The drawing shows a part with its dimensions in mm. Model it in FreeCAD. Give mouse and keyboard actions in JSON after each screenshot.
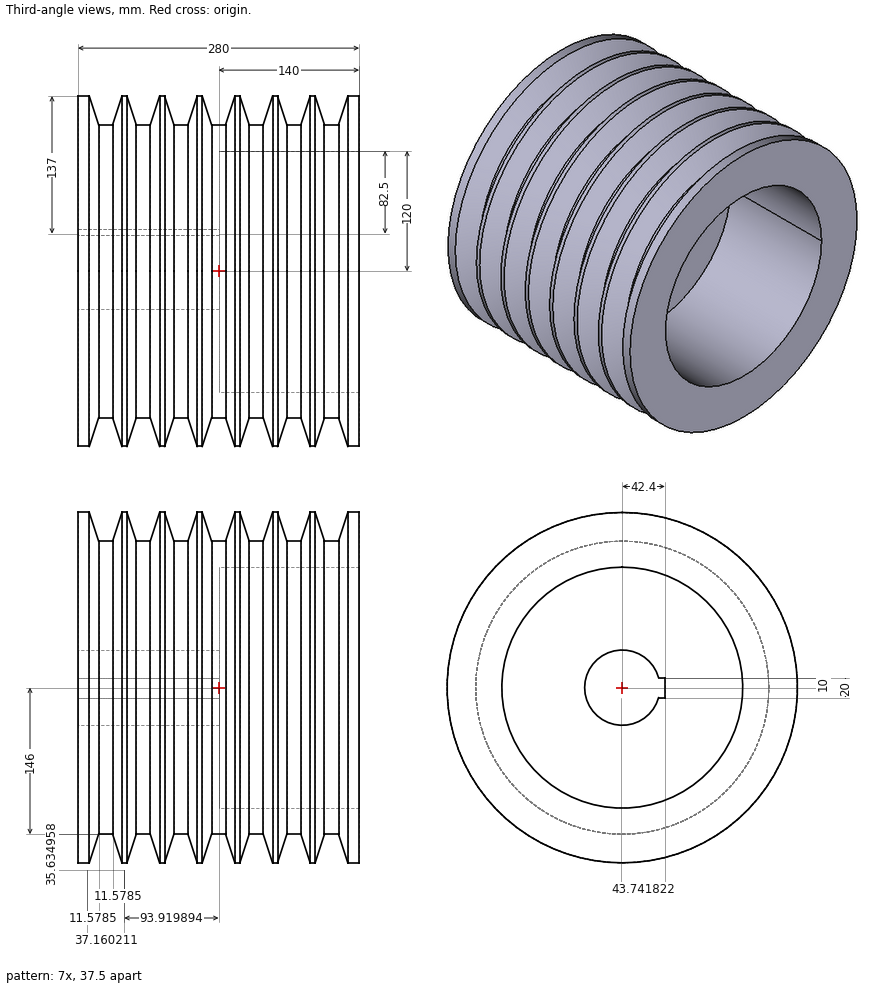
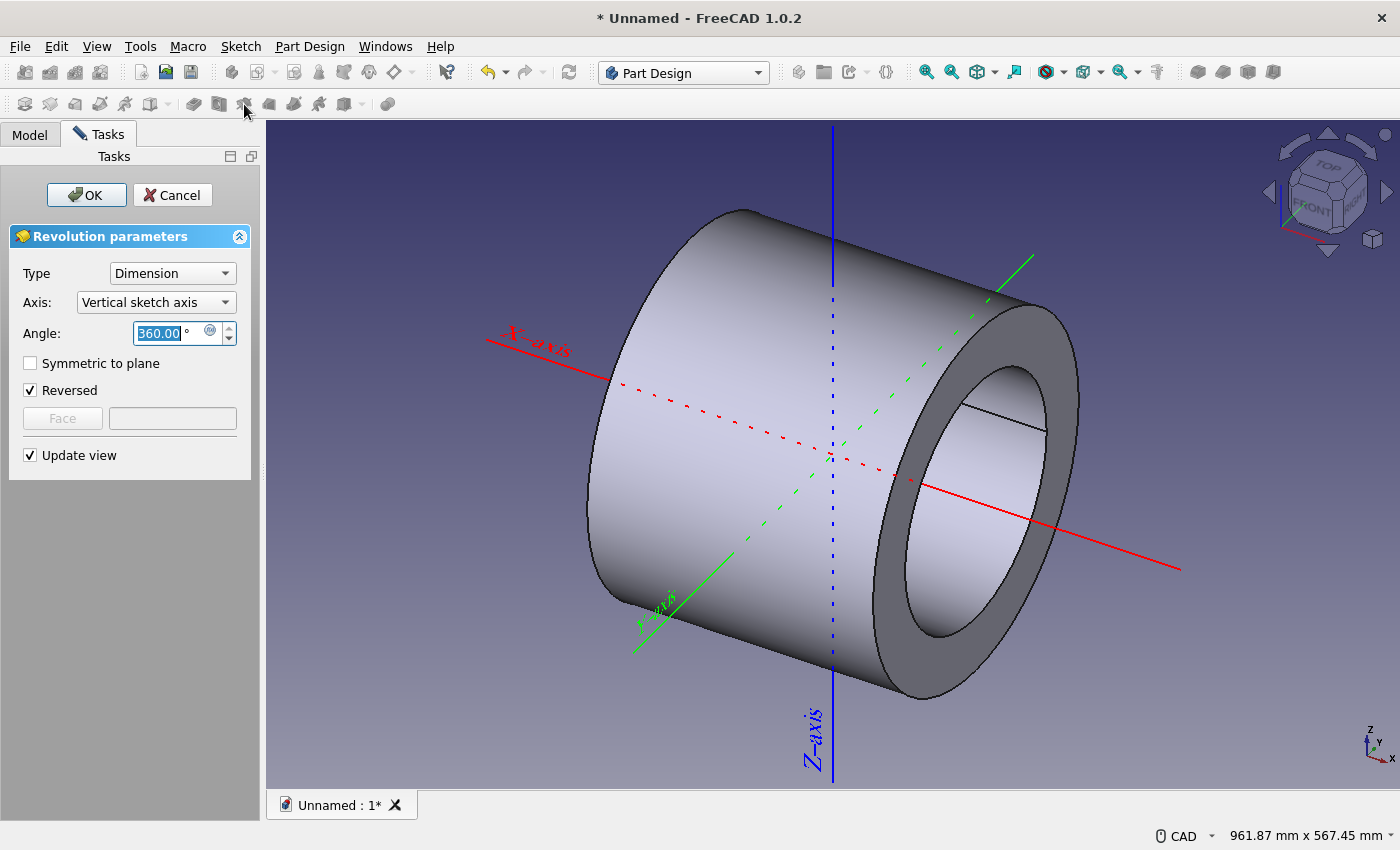
{"action": "left_click", "coordinate": [157, 302]}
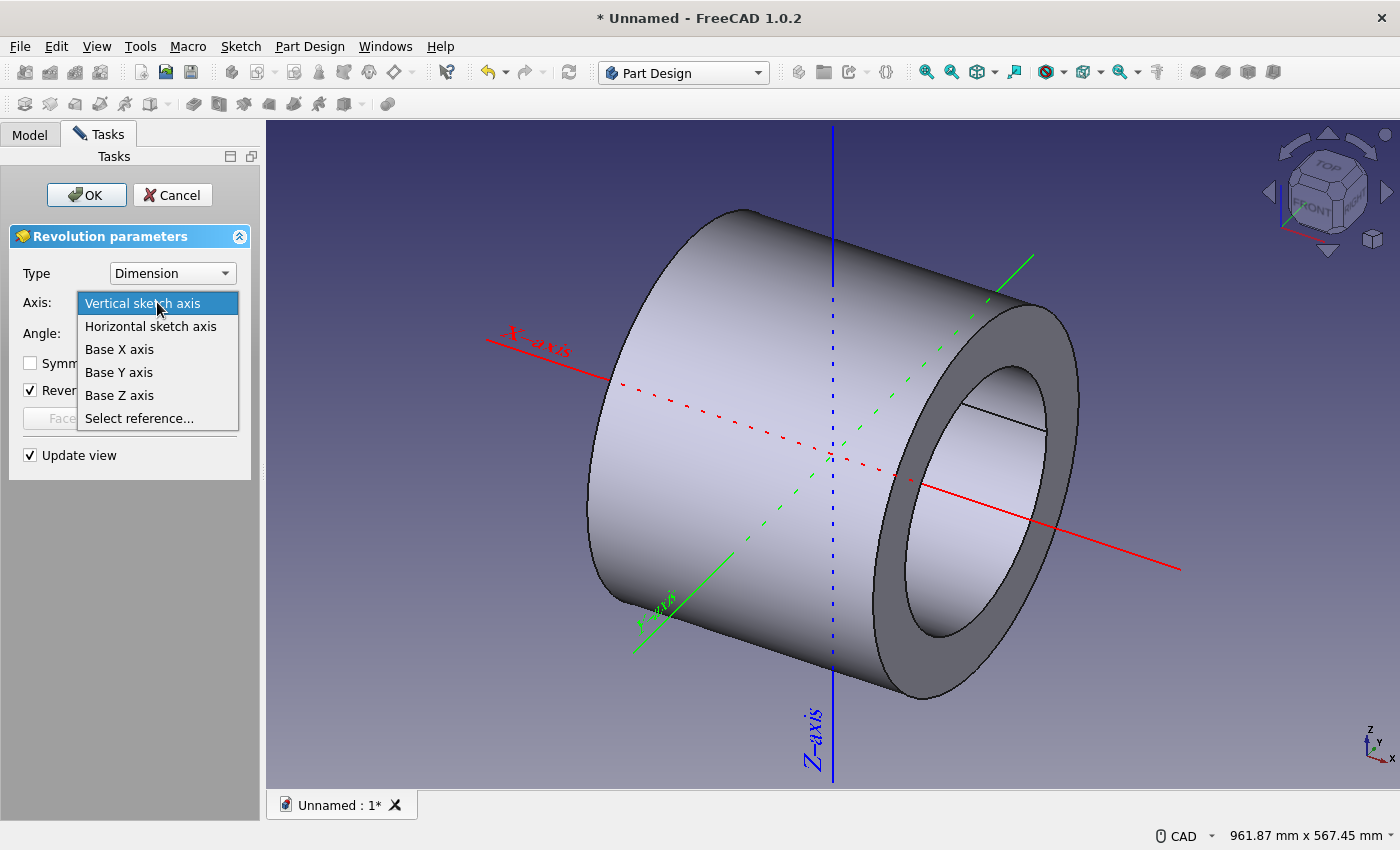
{"action": "left_click", "coordinate": [156, 326]}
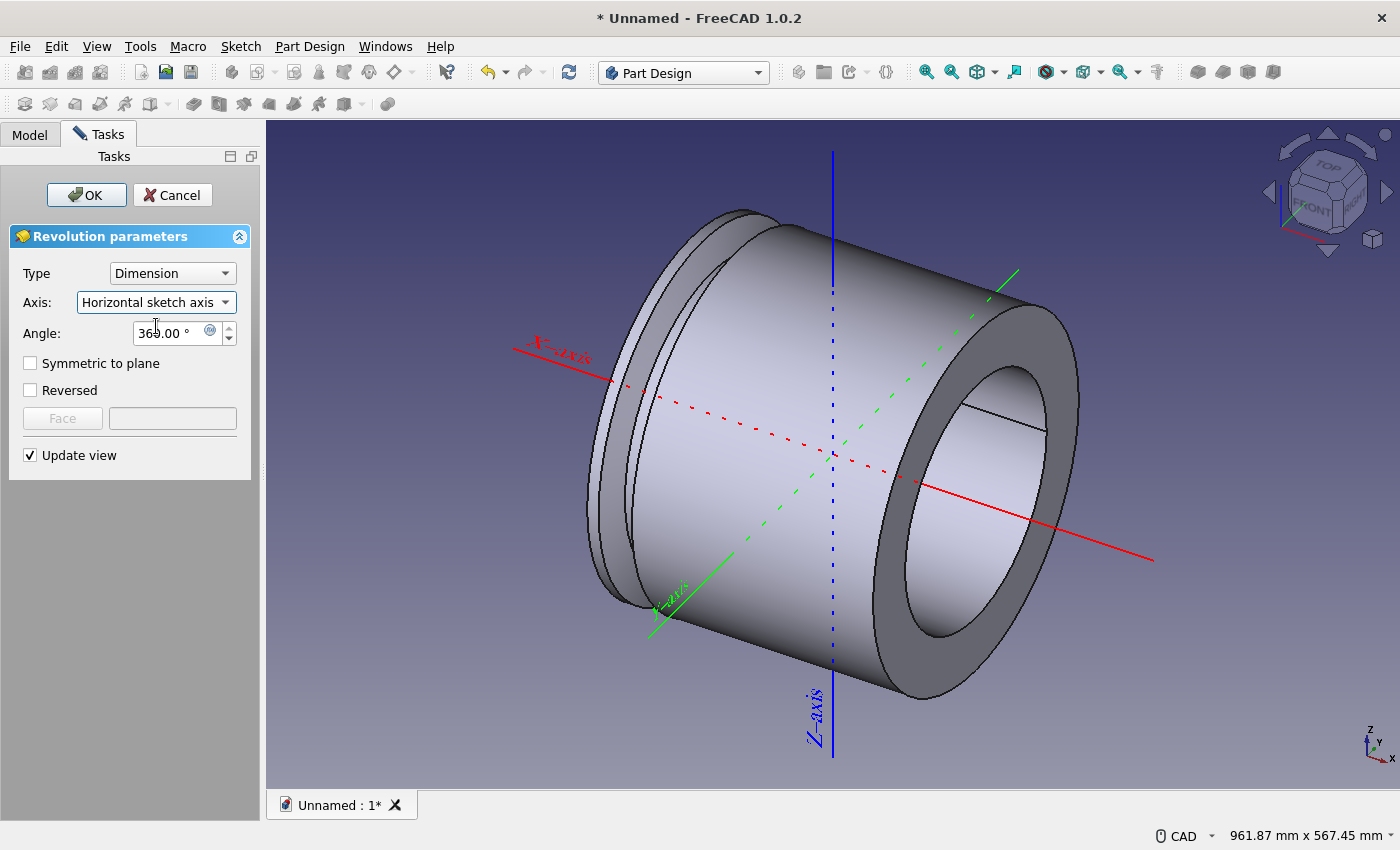
{"action": "left_click", "coordinate": [87, 195]}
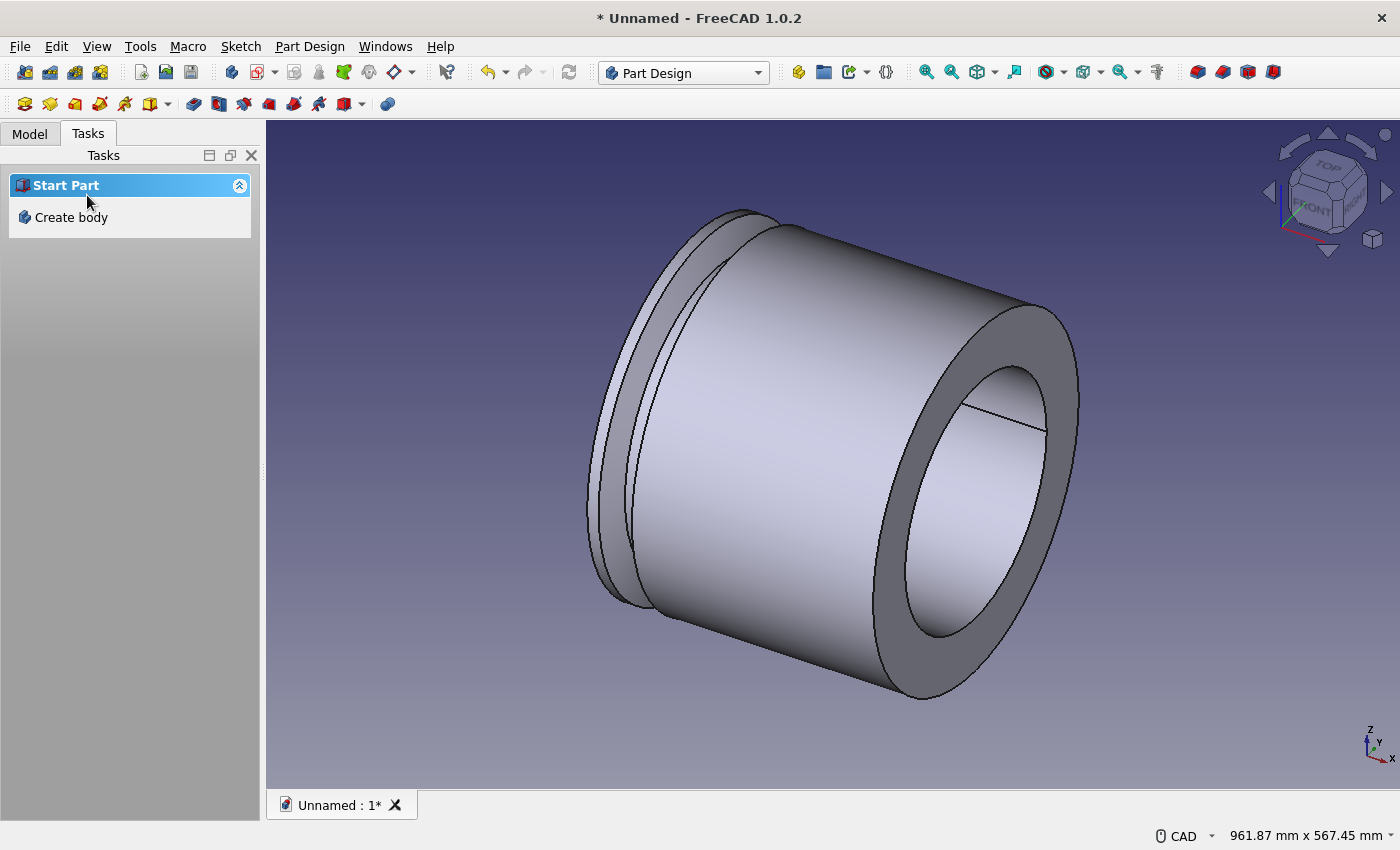
{"action": "key", "text": "6"}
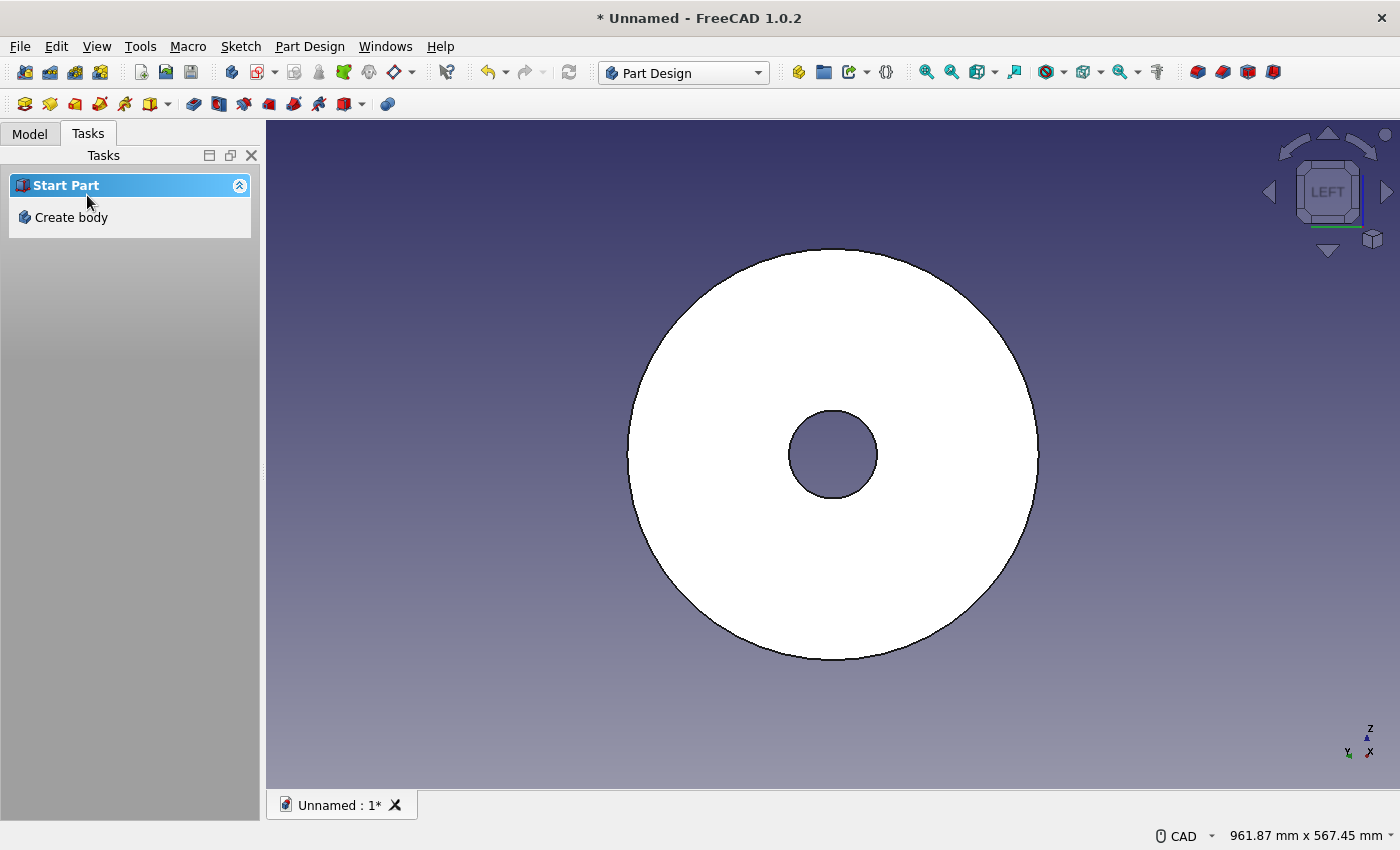
{"action": "left_click", "coordinate": [951, 512]}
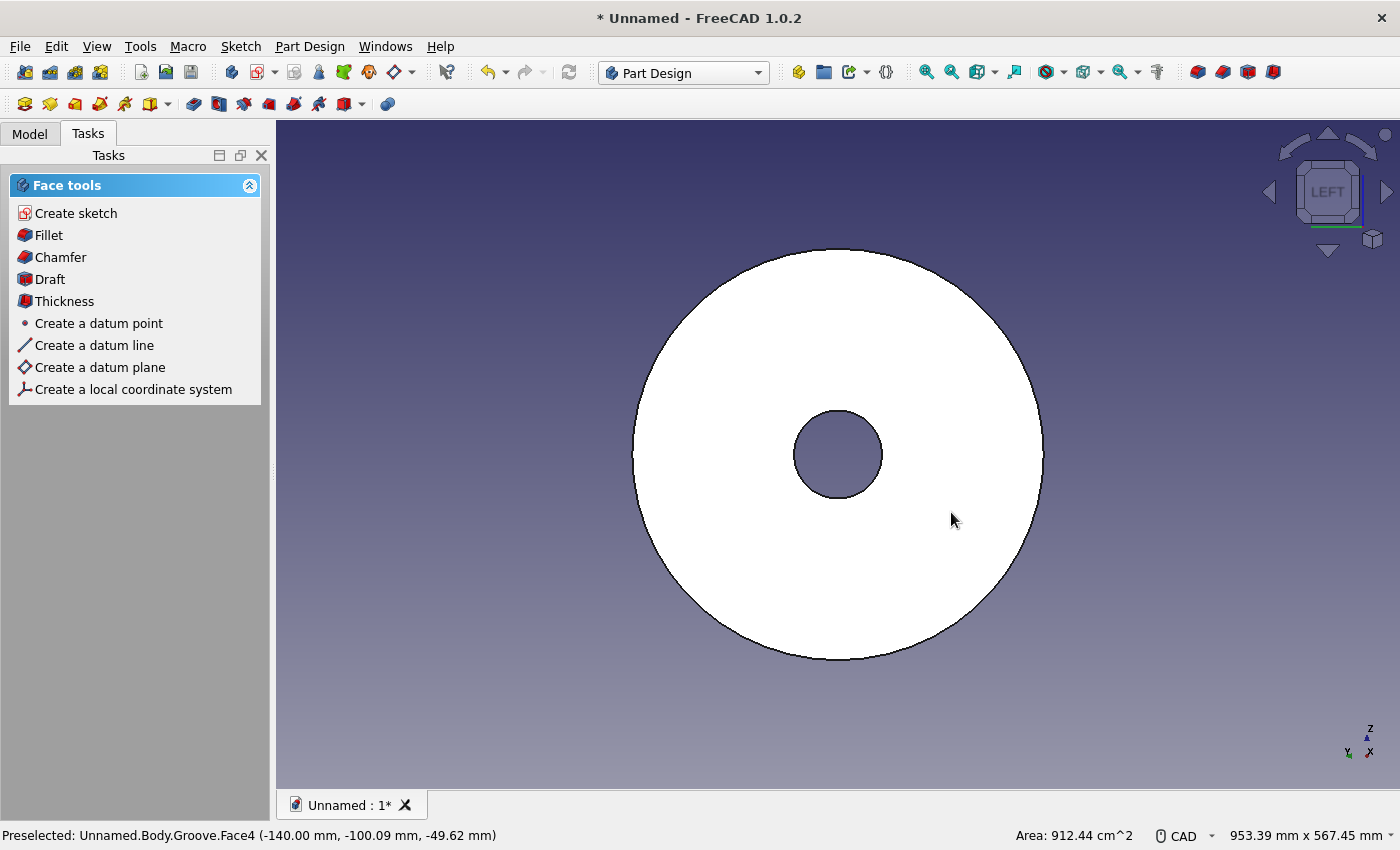
{"action": "left_click", "coordinate": [256, 72]}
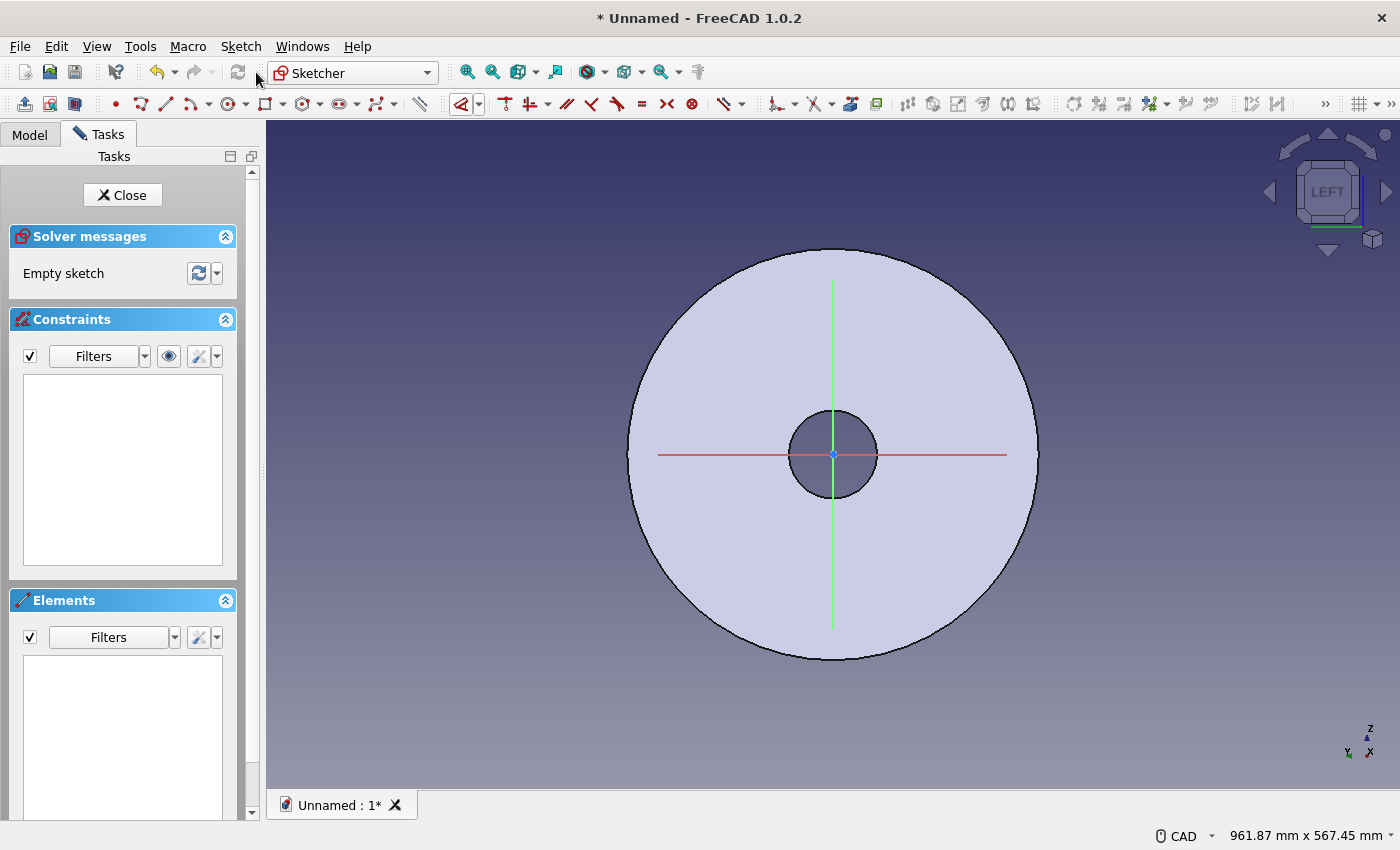
{"action": "scroll", "coordinate": [812, 455], "scroll_direction": "up", "scroll_amount": 13}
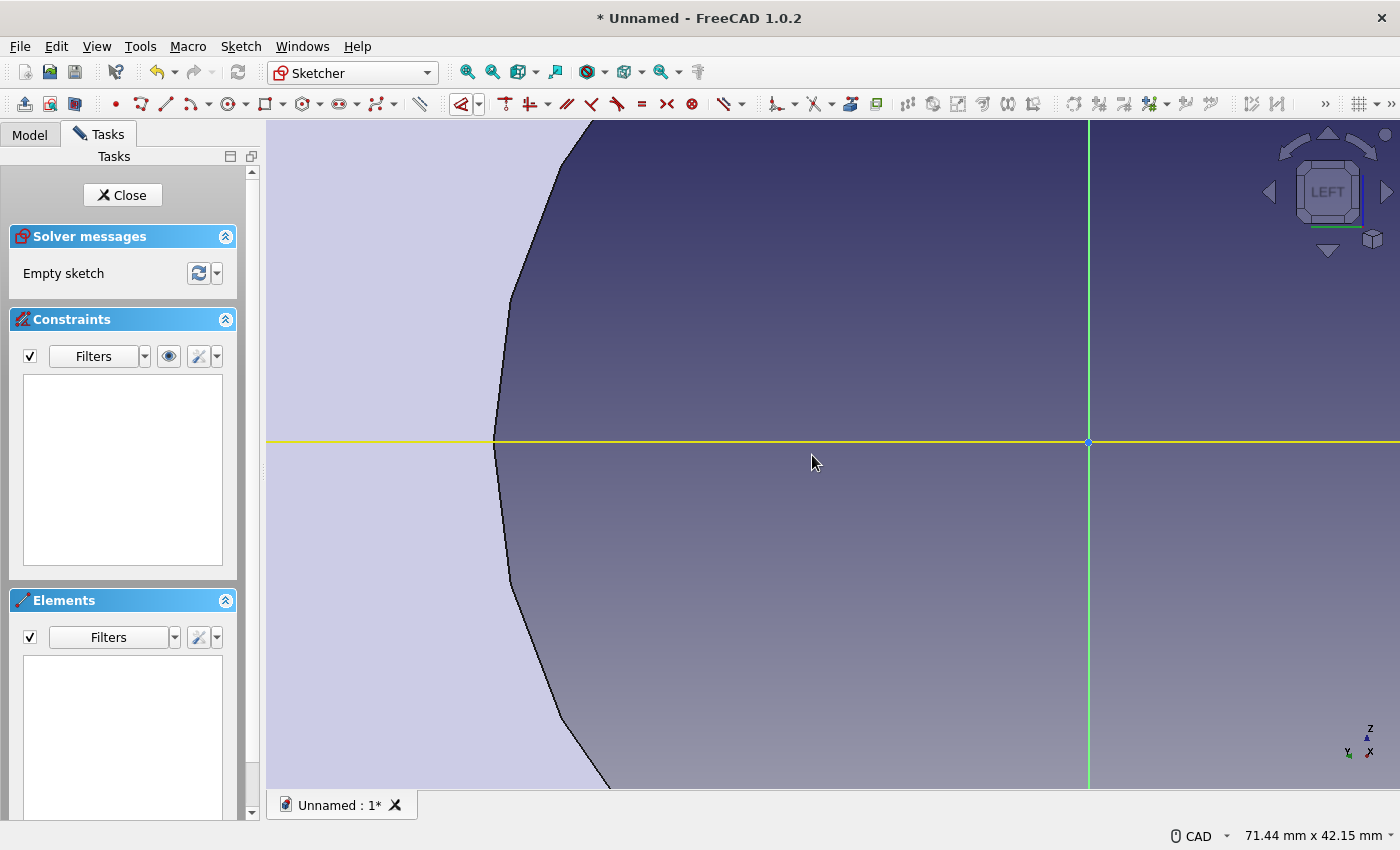
{"action": "left_click", "coordinate": [264, 104]}